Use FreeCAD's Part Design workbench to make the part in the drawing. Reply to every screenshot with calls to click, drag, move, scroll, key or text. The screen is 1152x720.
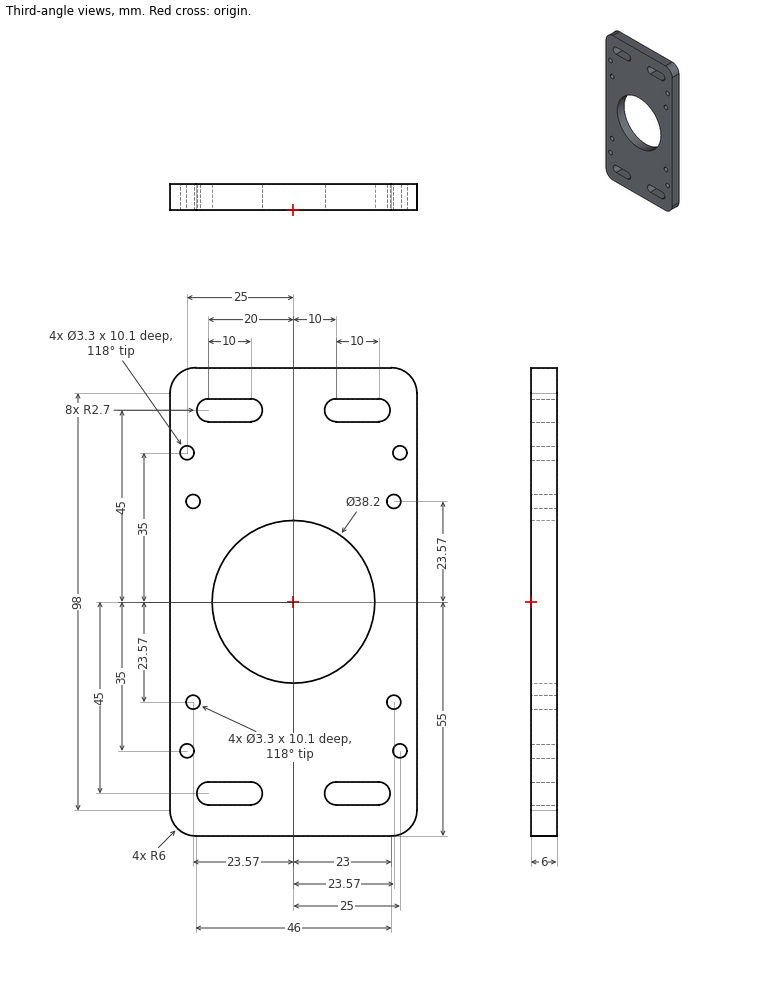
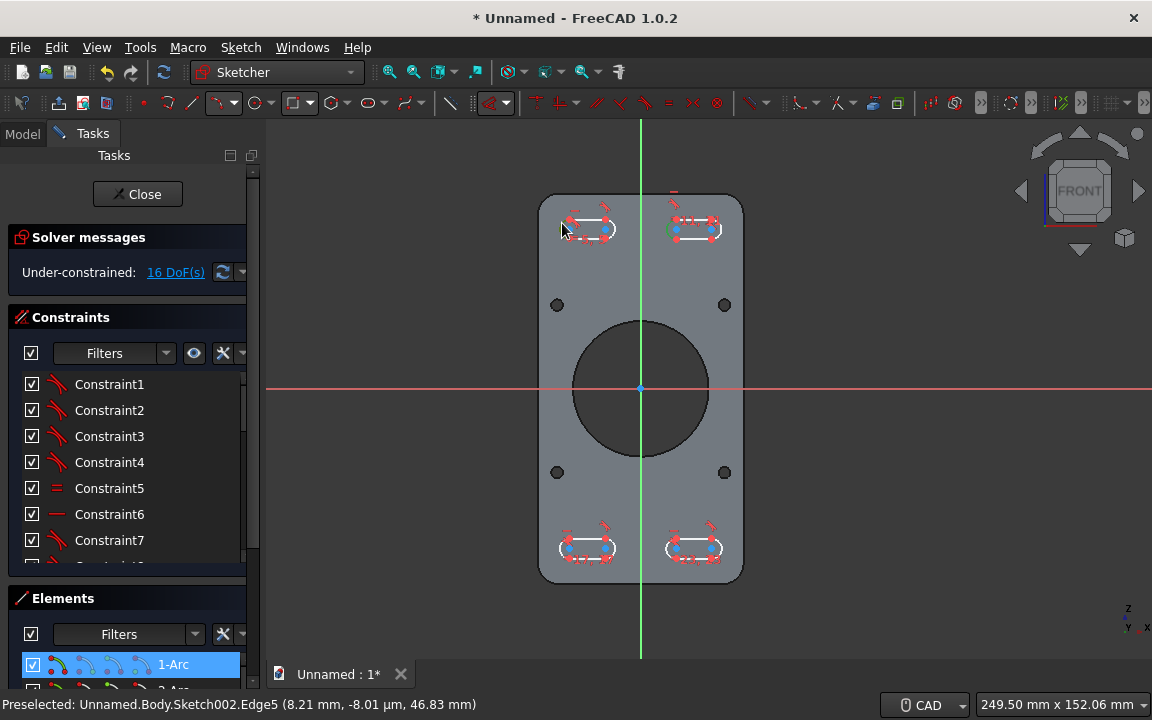
scroll(562, 543, up, 3)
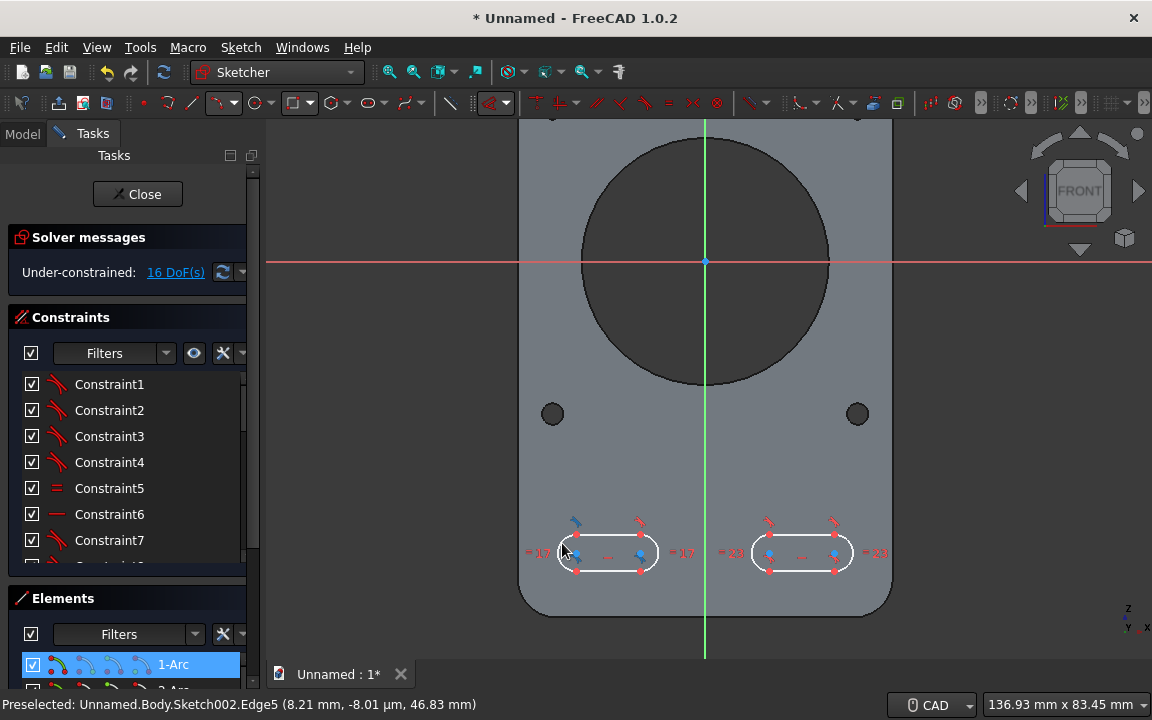
click(561, 542)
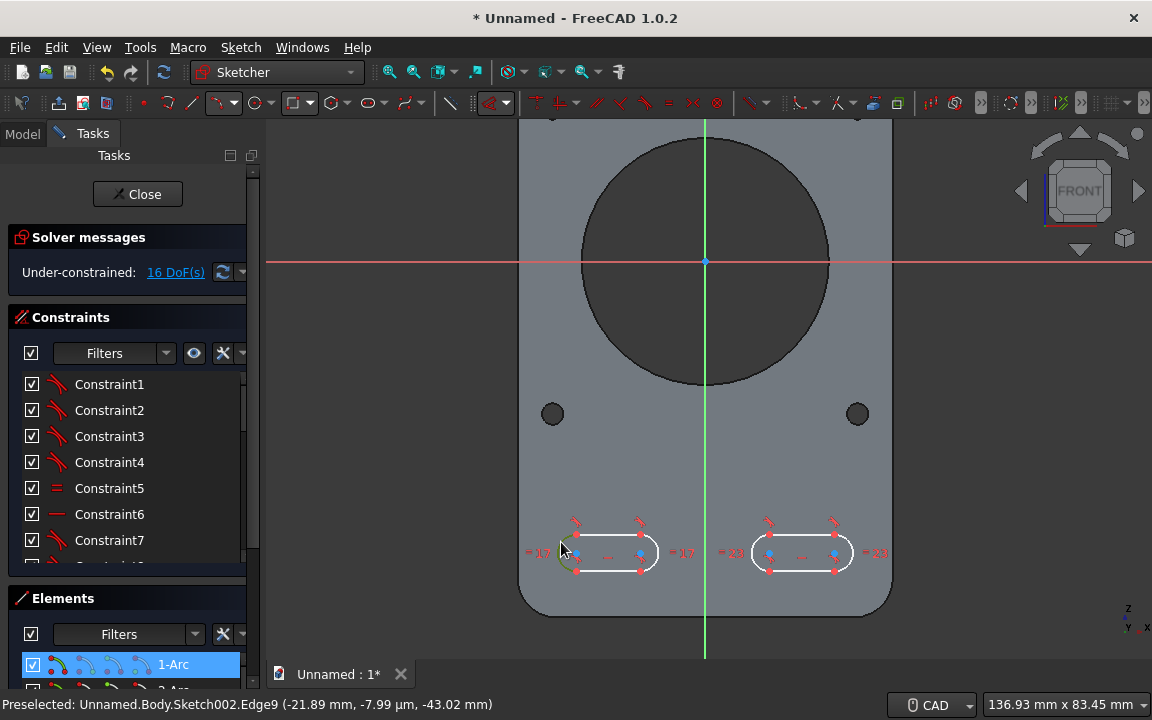
click(755, 542)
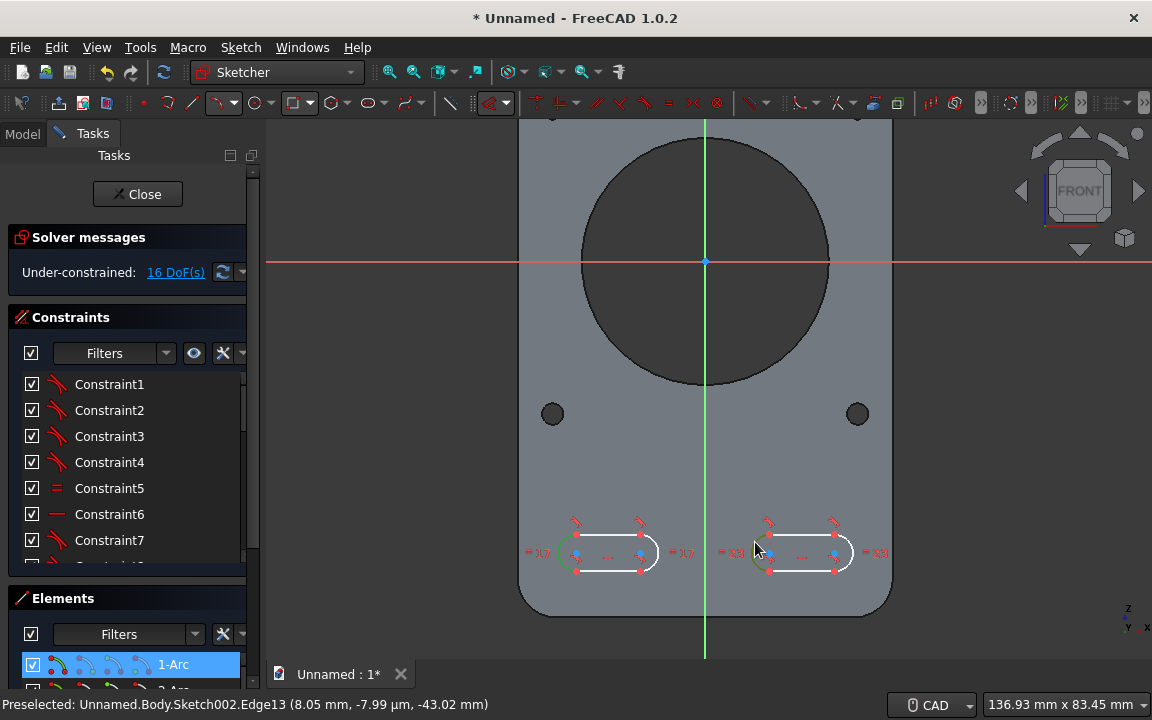
click(670, 104)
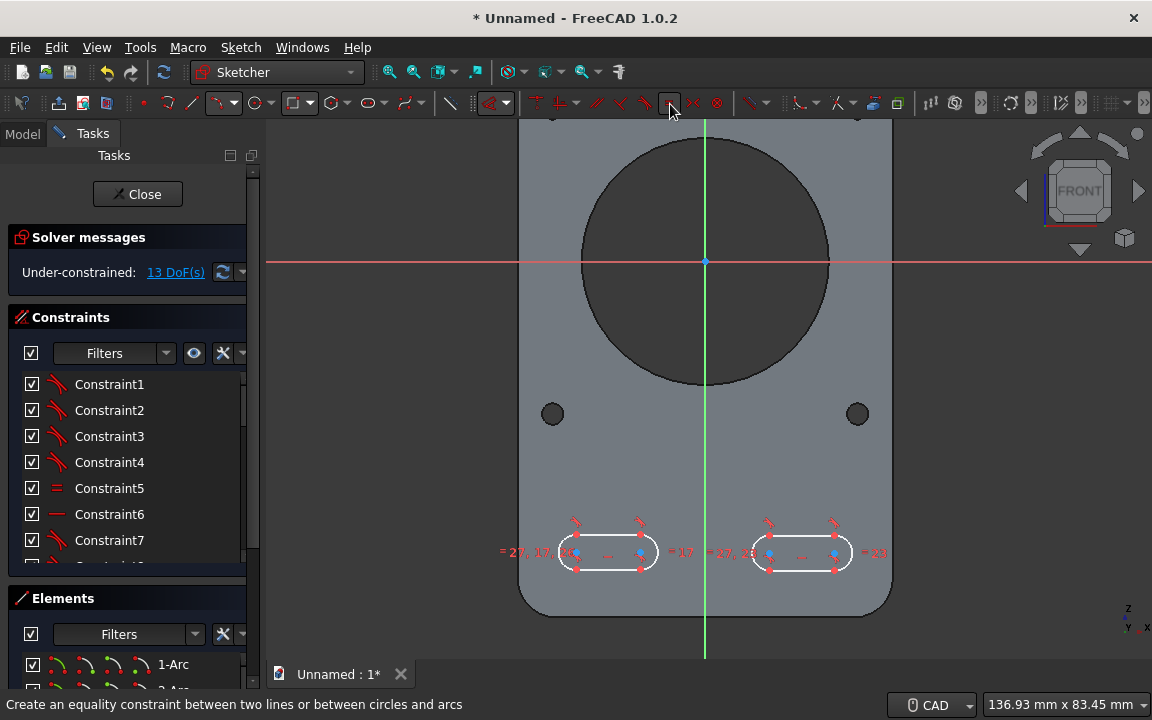
scroll(562, 544, down, 3)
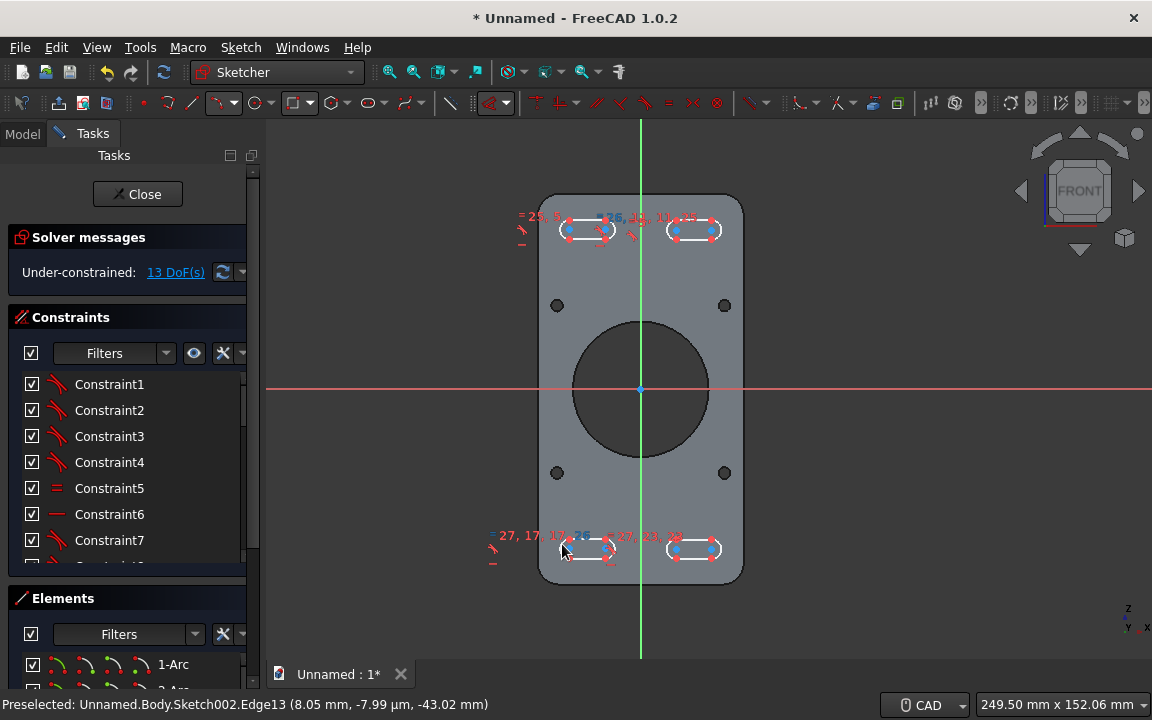
scroll(562, 224, up, 8)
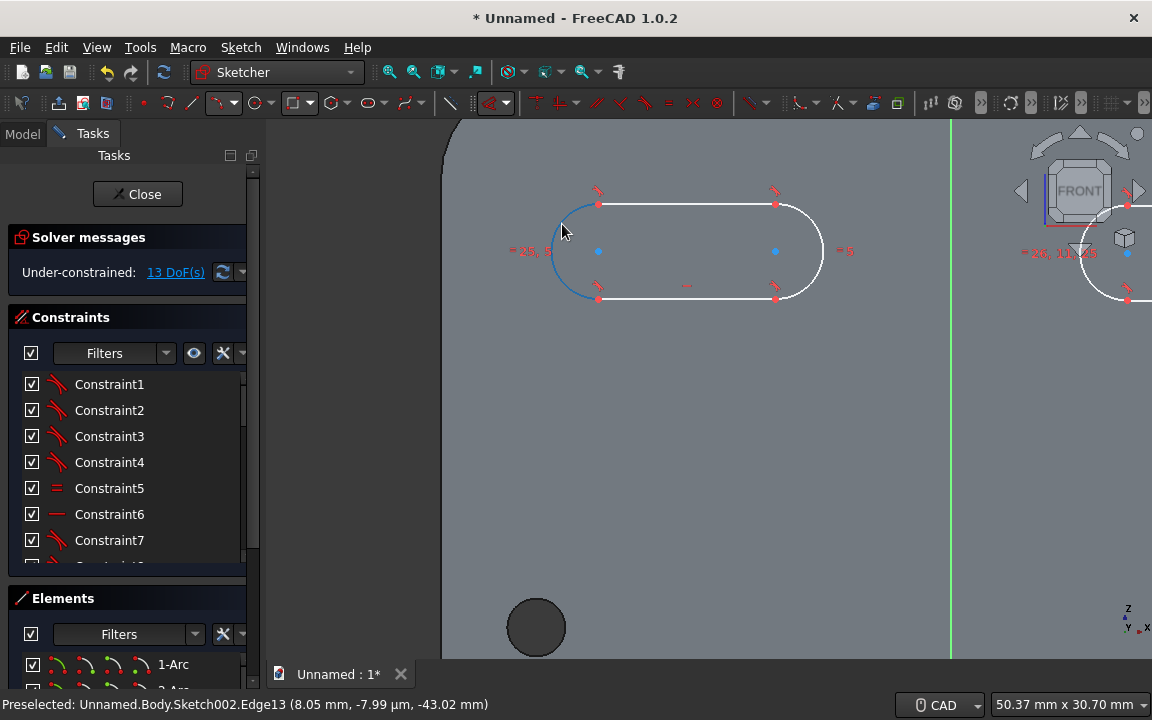
click(561, 224)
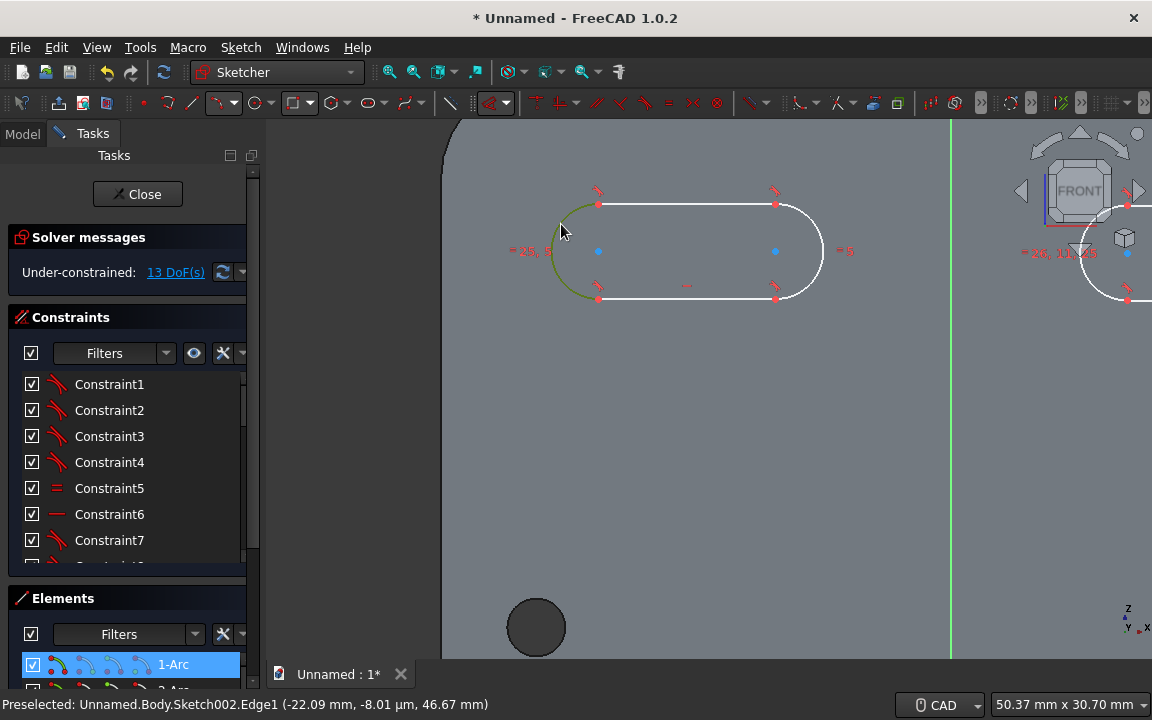
click(508, 104)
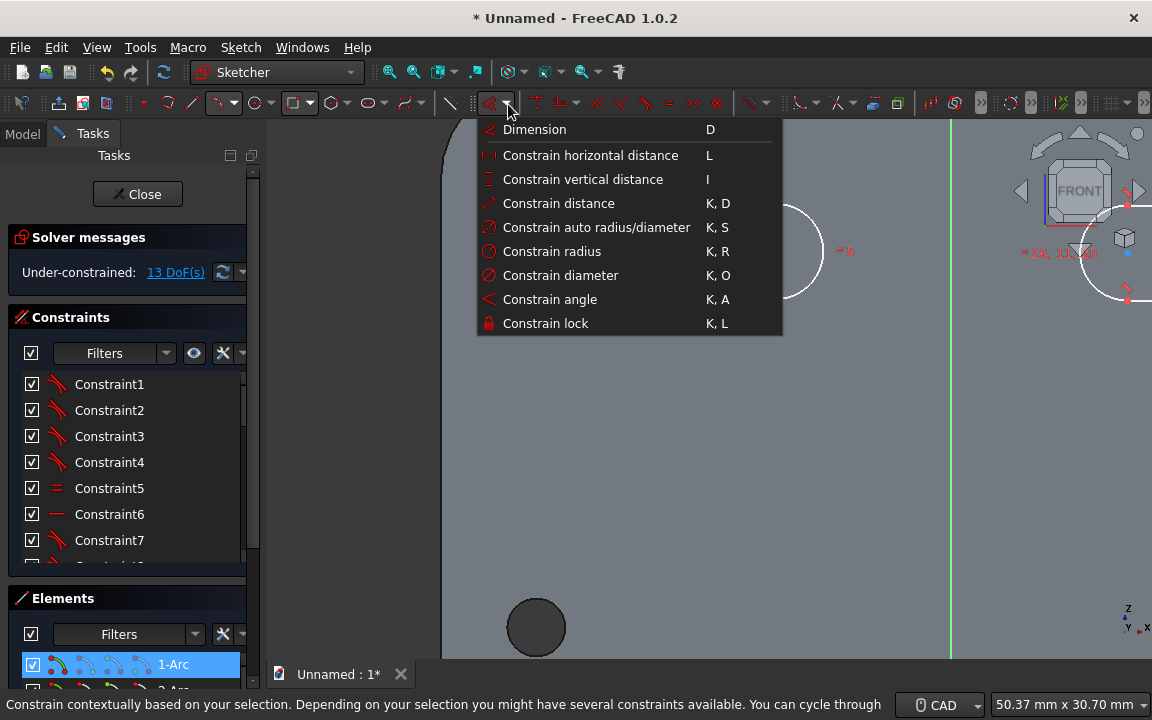
click(630, 251)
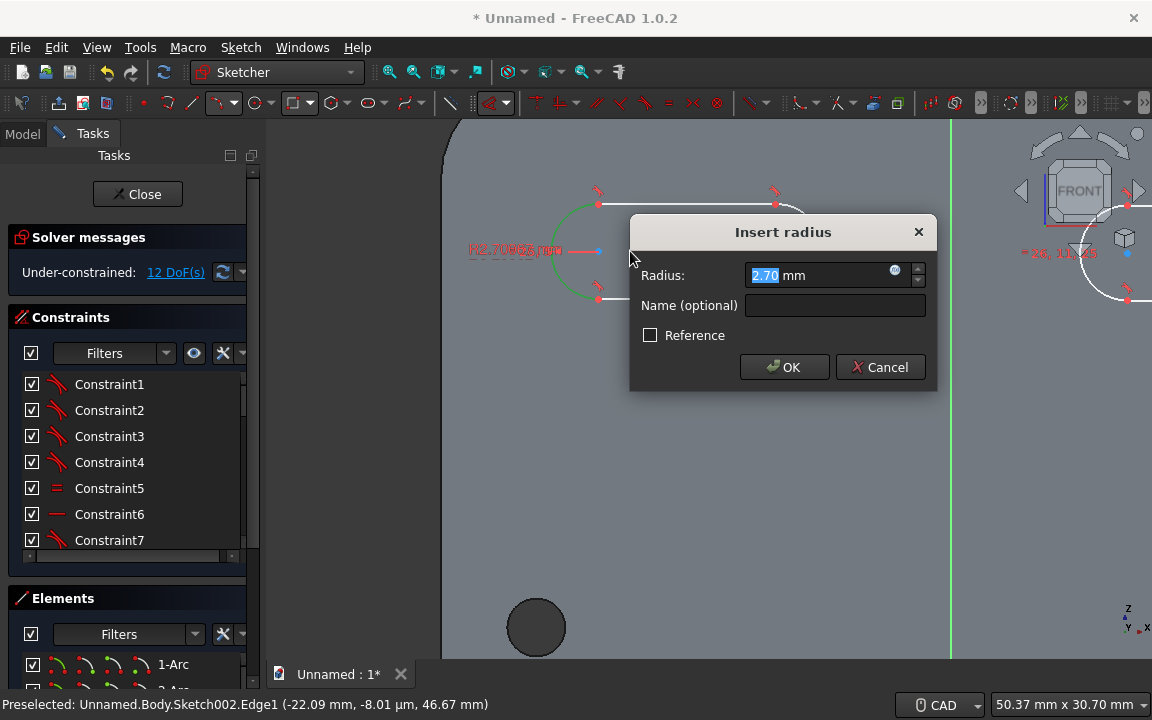
text(2.7)
key(Return)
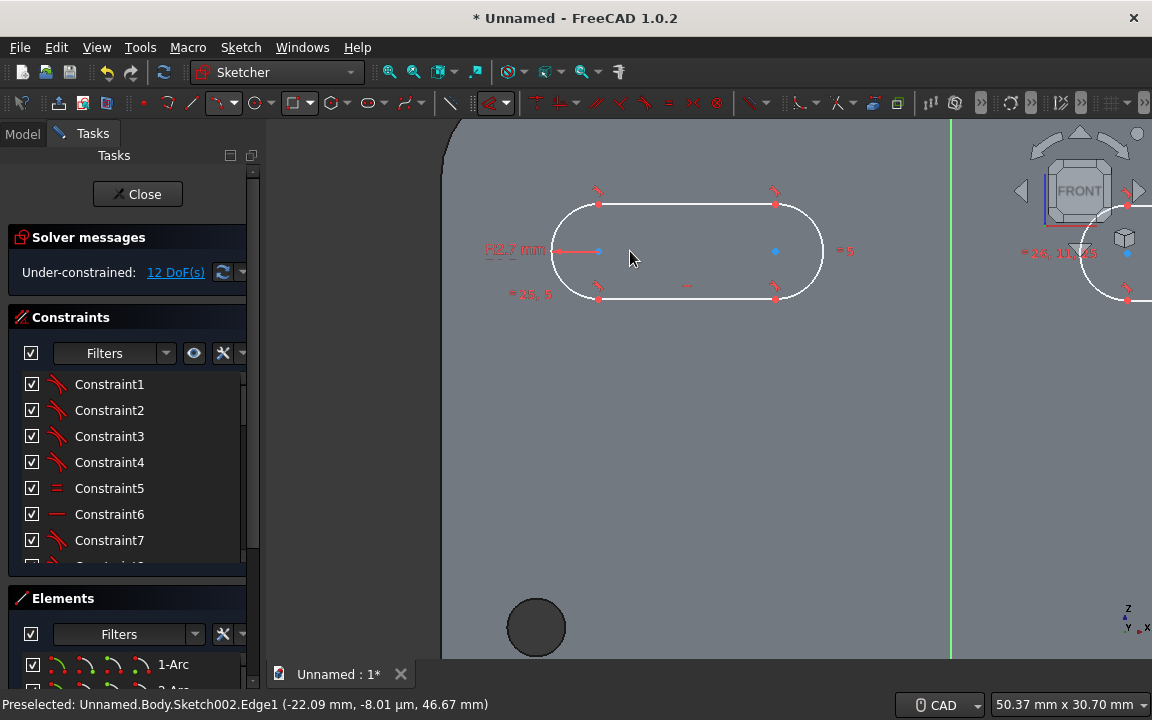
scroll(562, 224, down, 8)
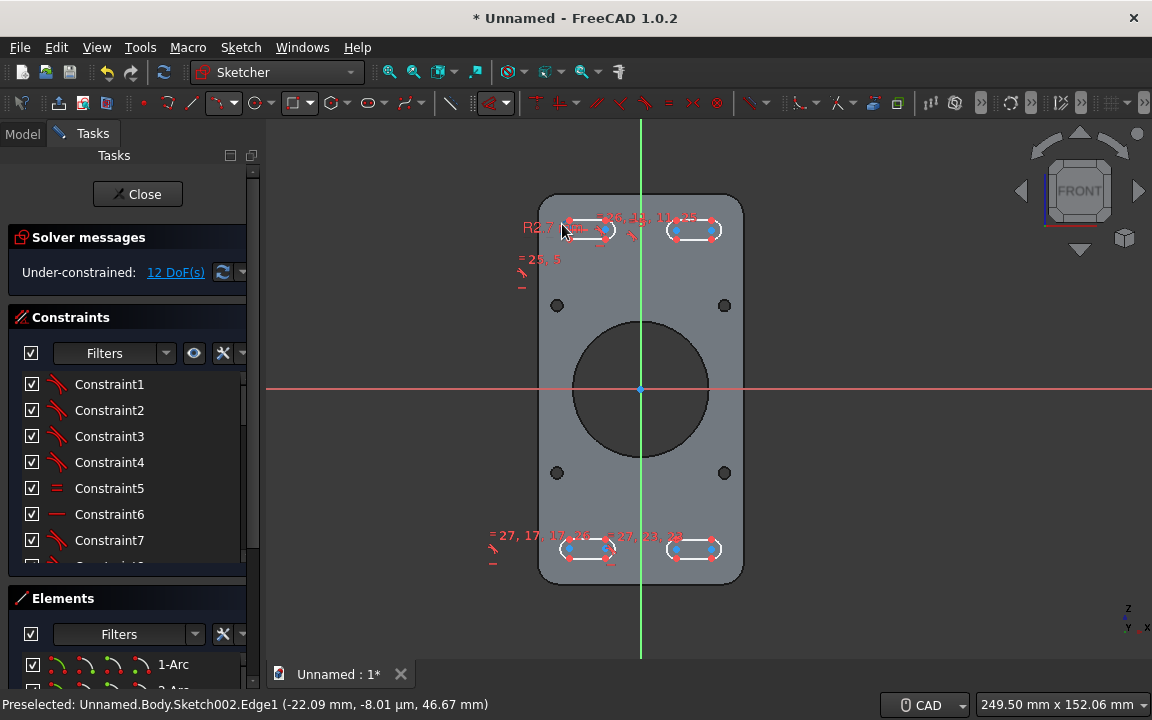
scroll(580, 220, up, 2)